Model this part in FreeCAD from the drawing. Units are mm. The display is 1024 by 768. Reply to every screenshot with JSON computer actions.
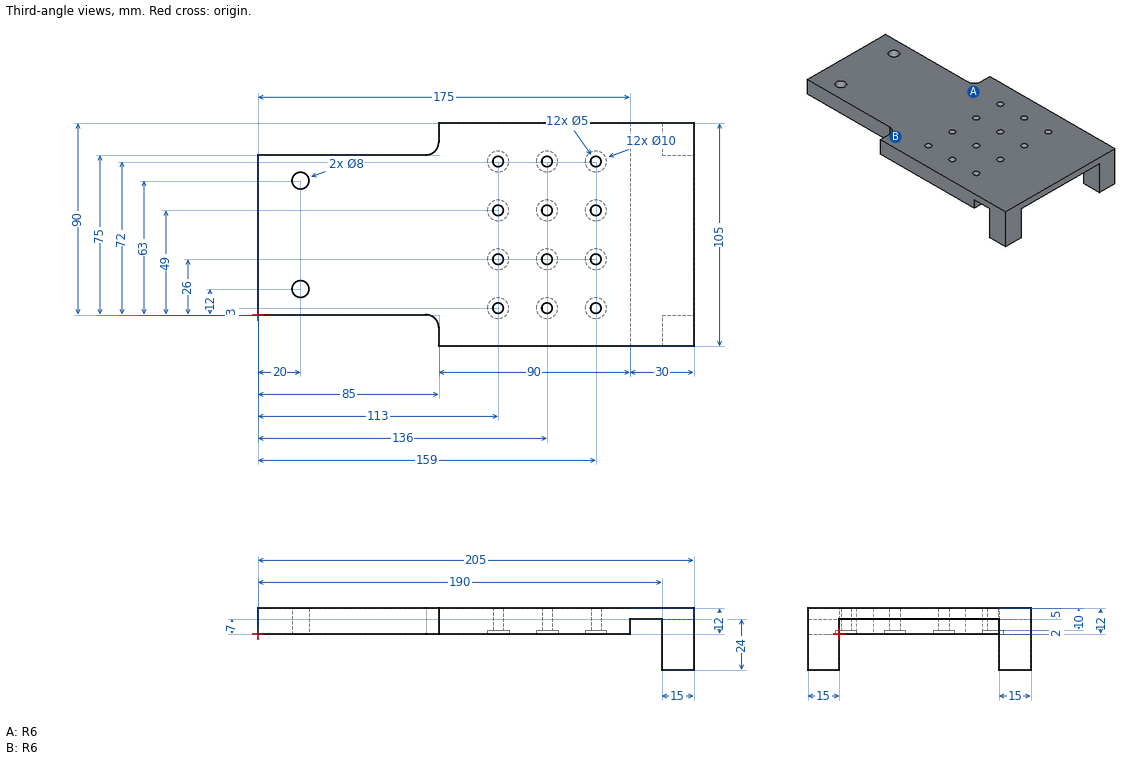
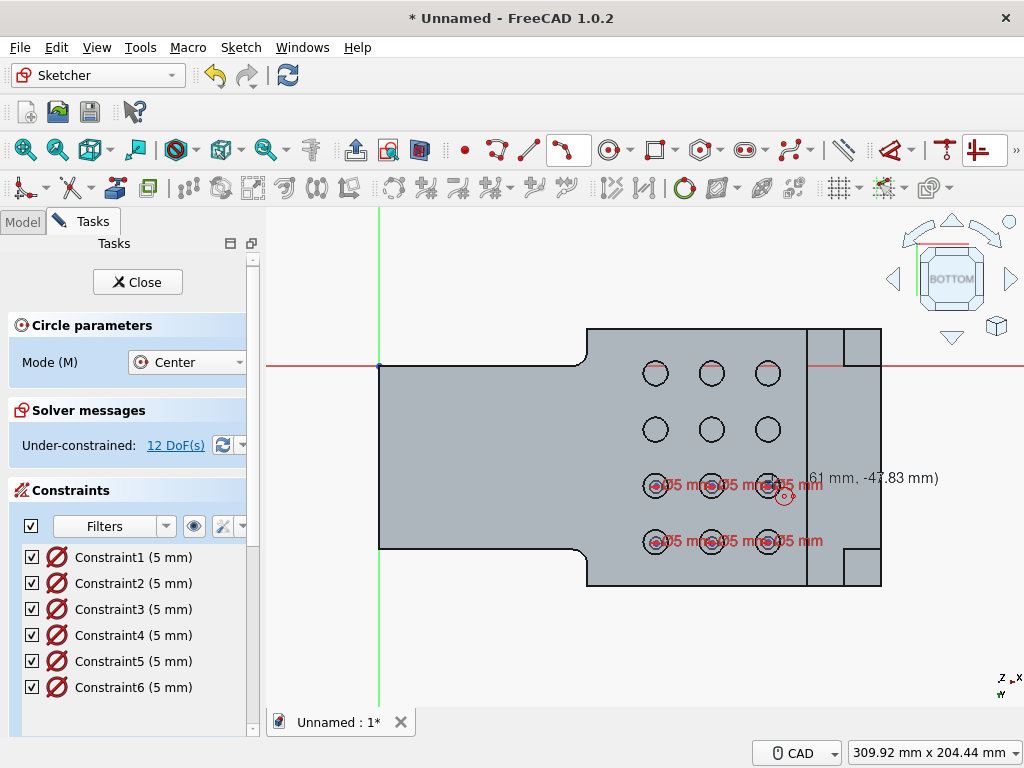
{"action": "scroll", "coordinate": [768, 430], "scroll_direction": "up", "scroll_amount": 7}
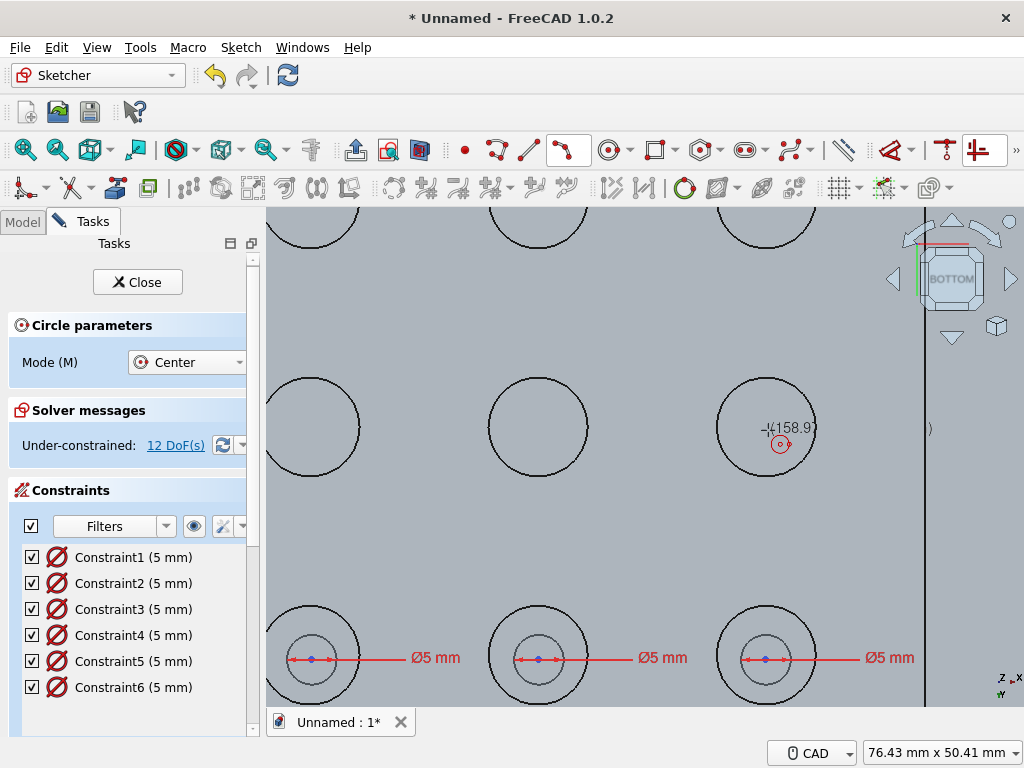
{"action": "scroll", "coordinate": [768, 430], "scroll_direction": "down", "scroll_amount": 7}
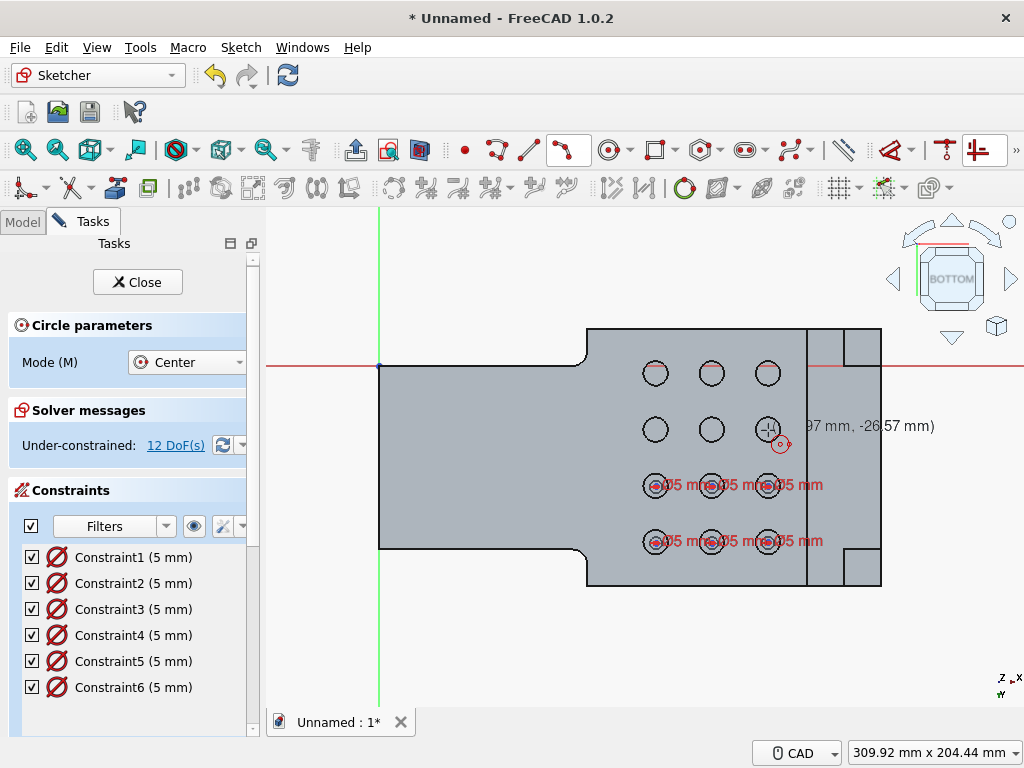
{"action": "left_click", "coordinate": [768, 430]}
{"action": "mouse_move", "coordinate": [772, 425]}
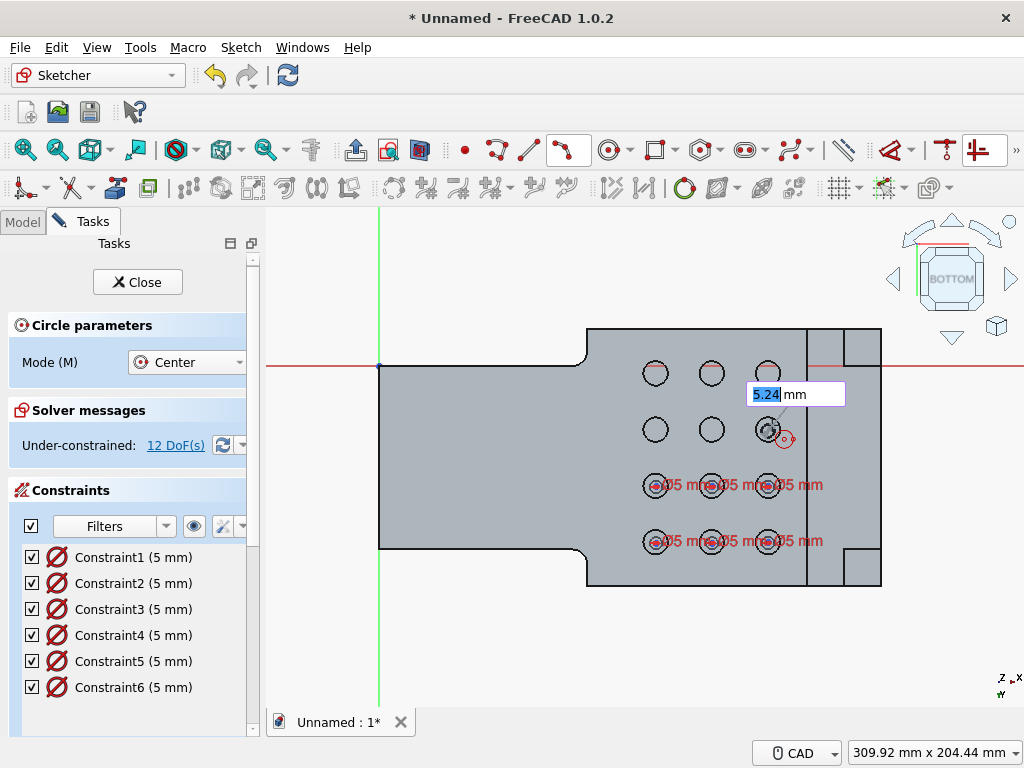
{"action": "type", "text": "5"}
{"action": "key", "text": "Return"}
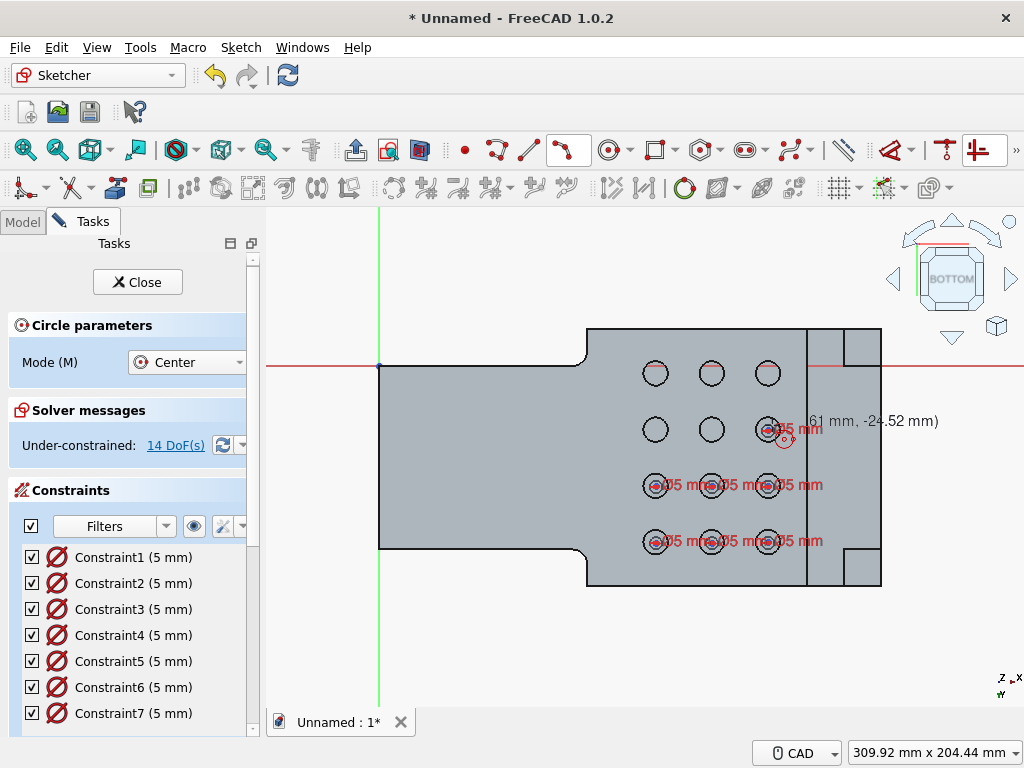
{"action": "scroll", "coordinate": [712, 430], "scroll_direction": "up", "scroll_amount": 7}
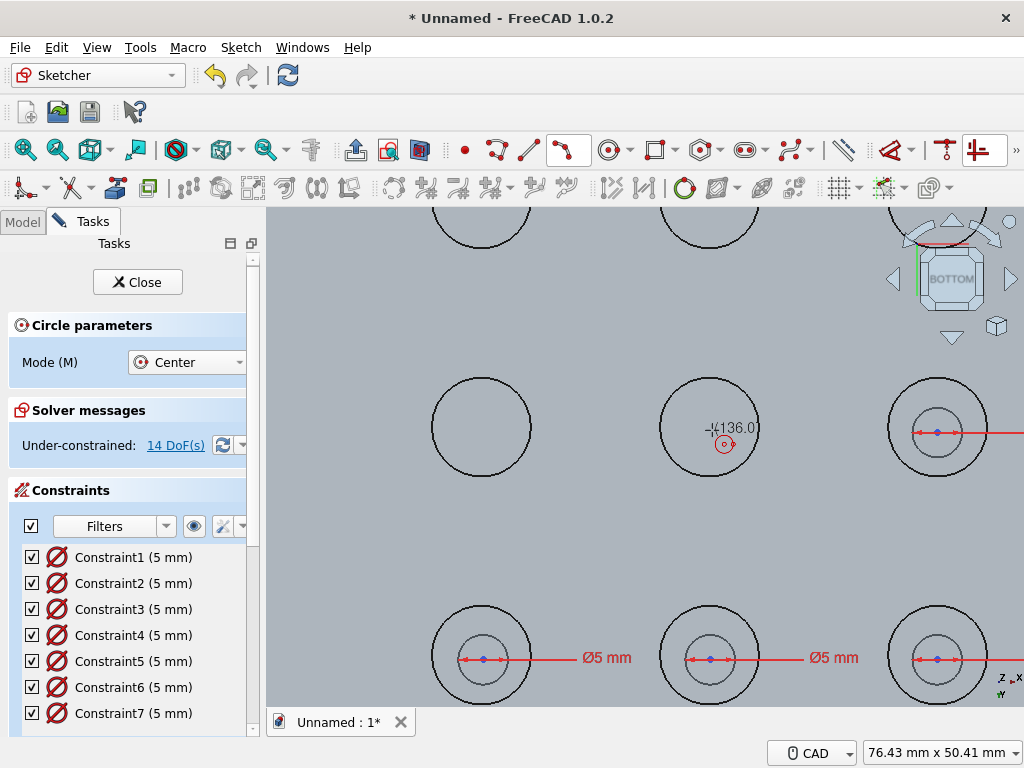
{"action": "scroll", "coordinate": [712, 430], "scroll_direction": "down", "scroll_amount": 7}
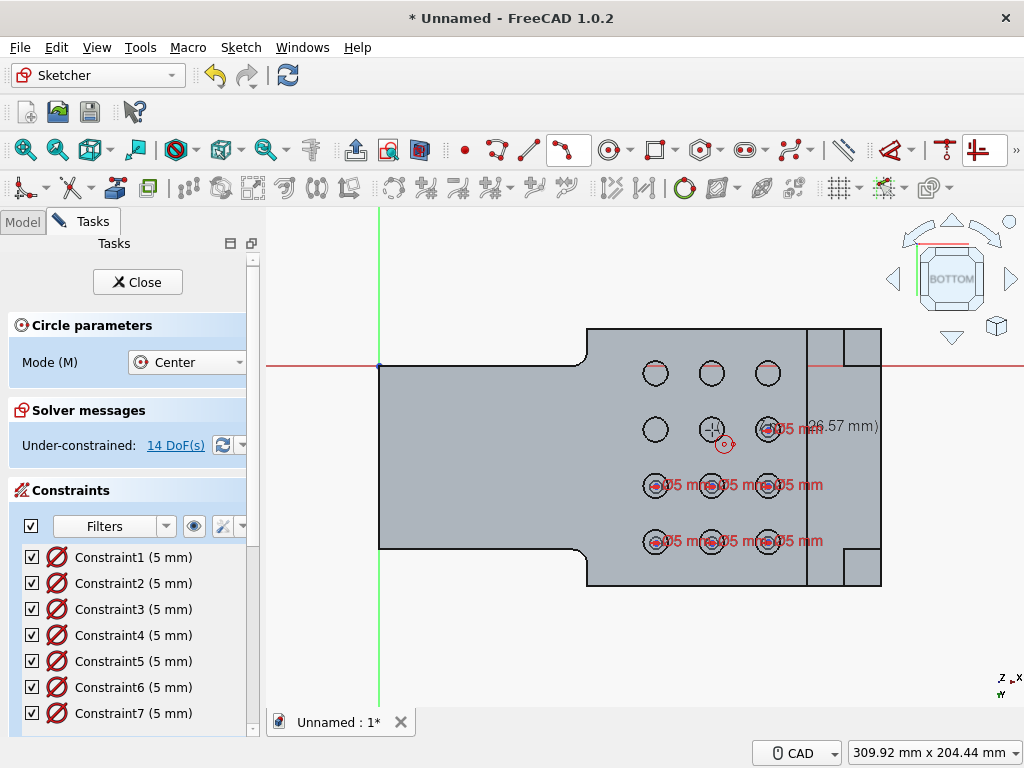
{"action": "left_click", "coordinate": [712, 430]}
{"action": "mouse_move", "coordinate": [716, 425]}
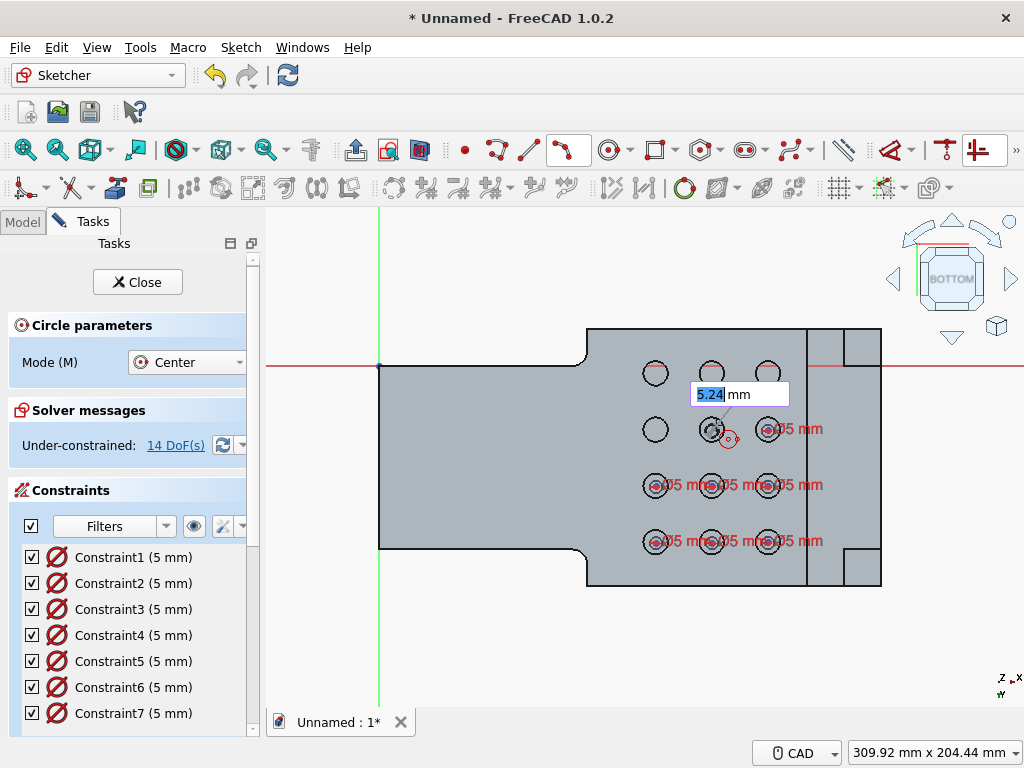
{"action": "type", "text": "5"}
{"action": "key", "text": "Return"}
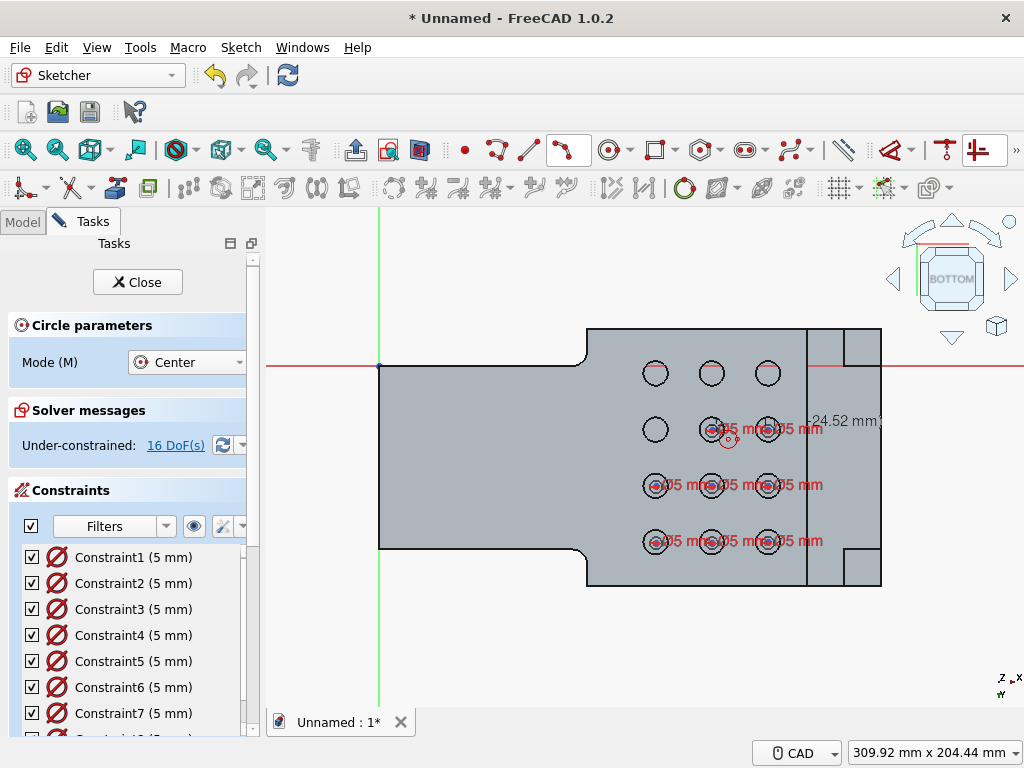
{"action": "scroll", "coordinate": [656, 430], "scroll_direction": "up", "scroll_amount": 7}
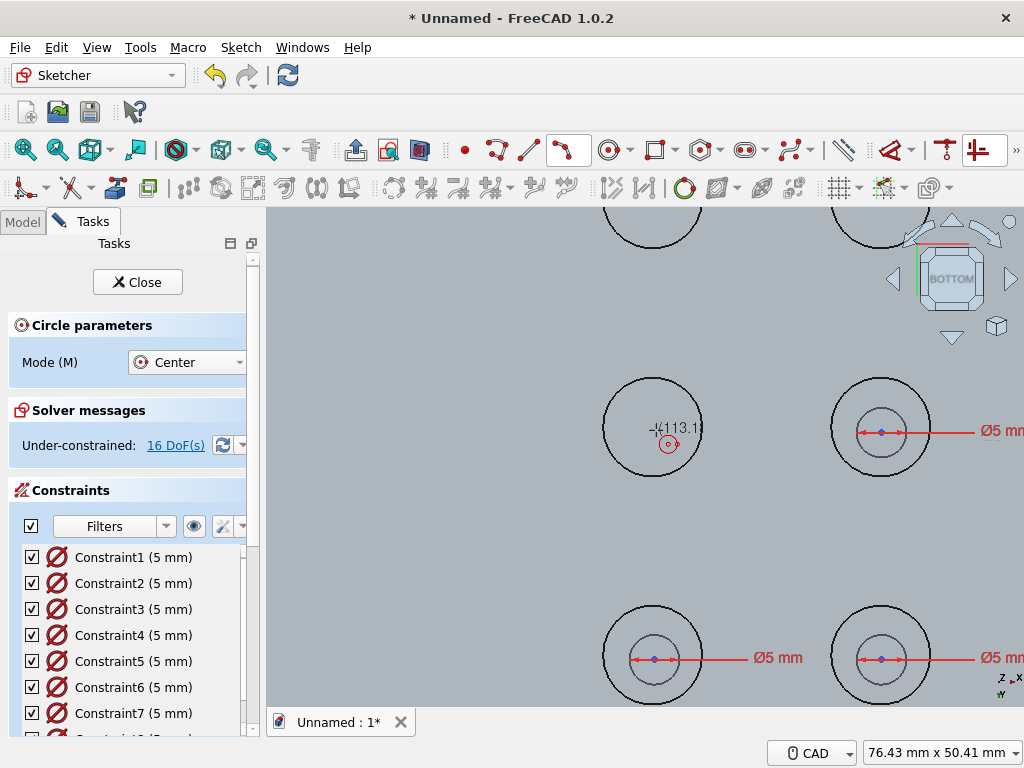
{"action": "scroll", "coordinate": [656, 430], "scroll_direction": "down", "scroll_amount": 7}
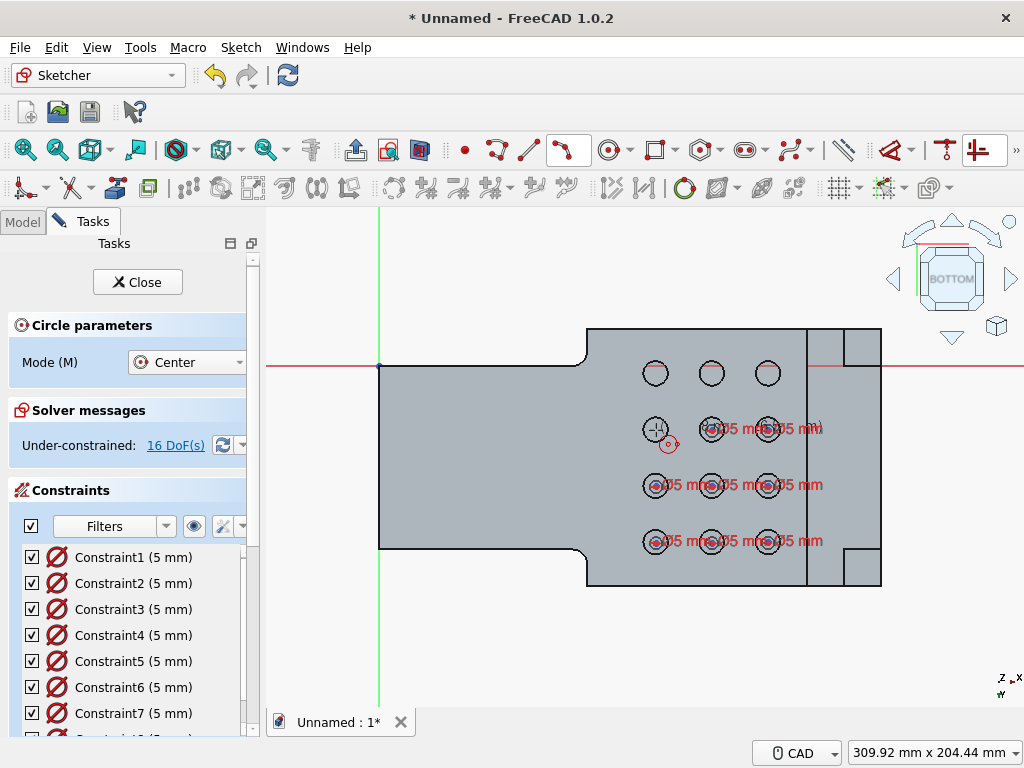
{"action": "left_click", "coordinate": [656, 430]}
{"action": "mouse_move", "coordinate": [660, 425]}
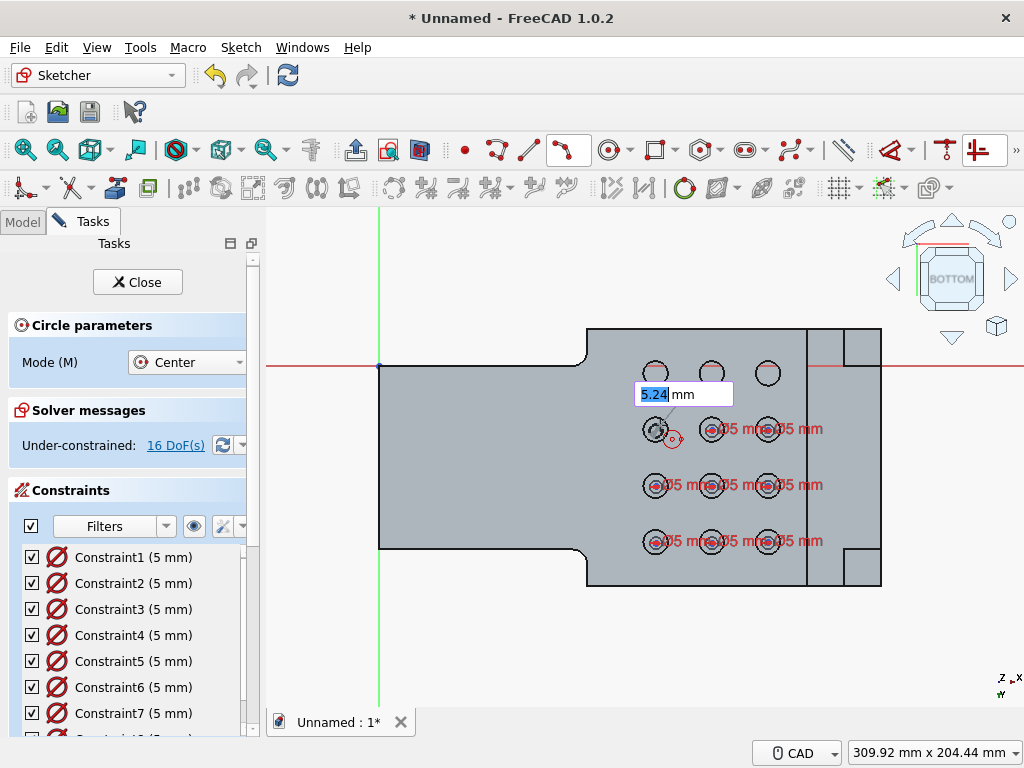
{"action": "type", "text": "5"}
{"action": "key", "text": "Return"}